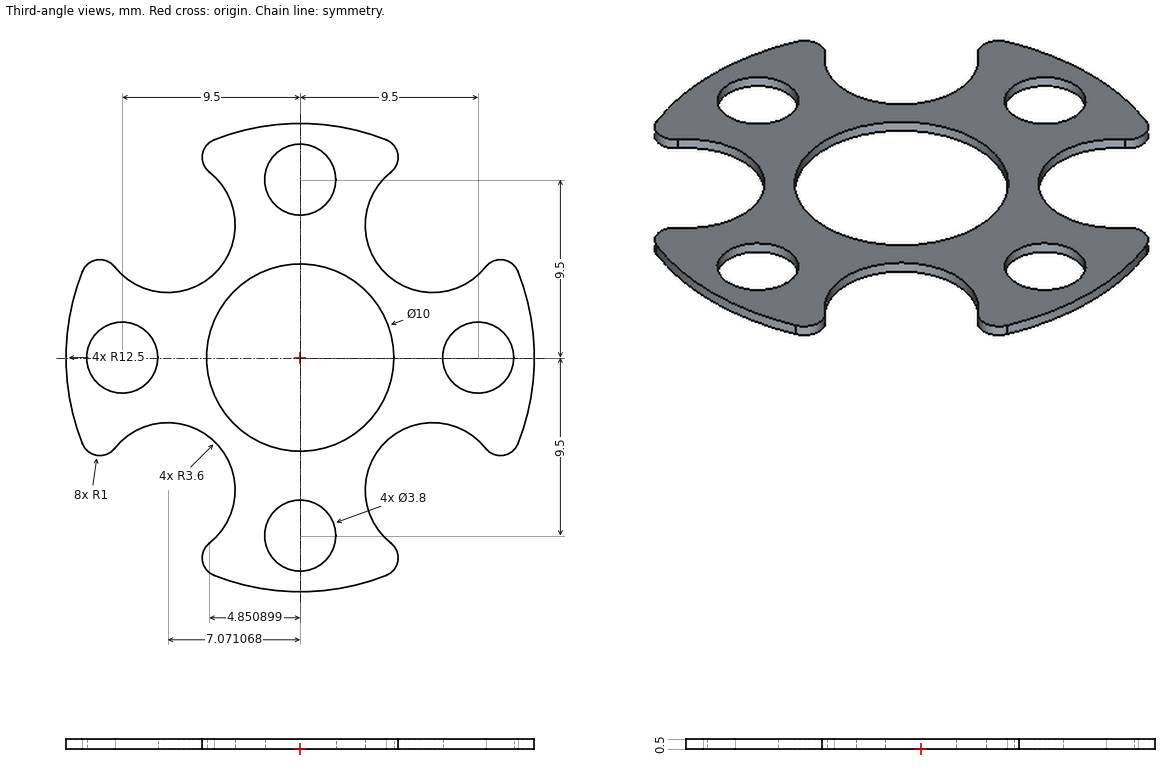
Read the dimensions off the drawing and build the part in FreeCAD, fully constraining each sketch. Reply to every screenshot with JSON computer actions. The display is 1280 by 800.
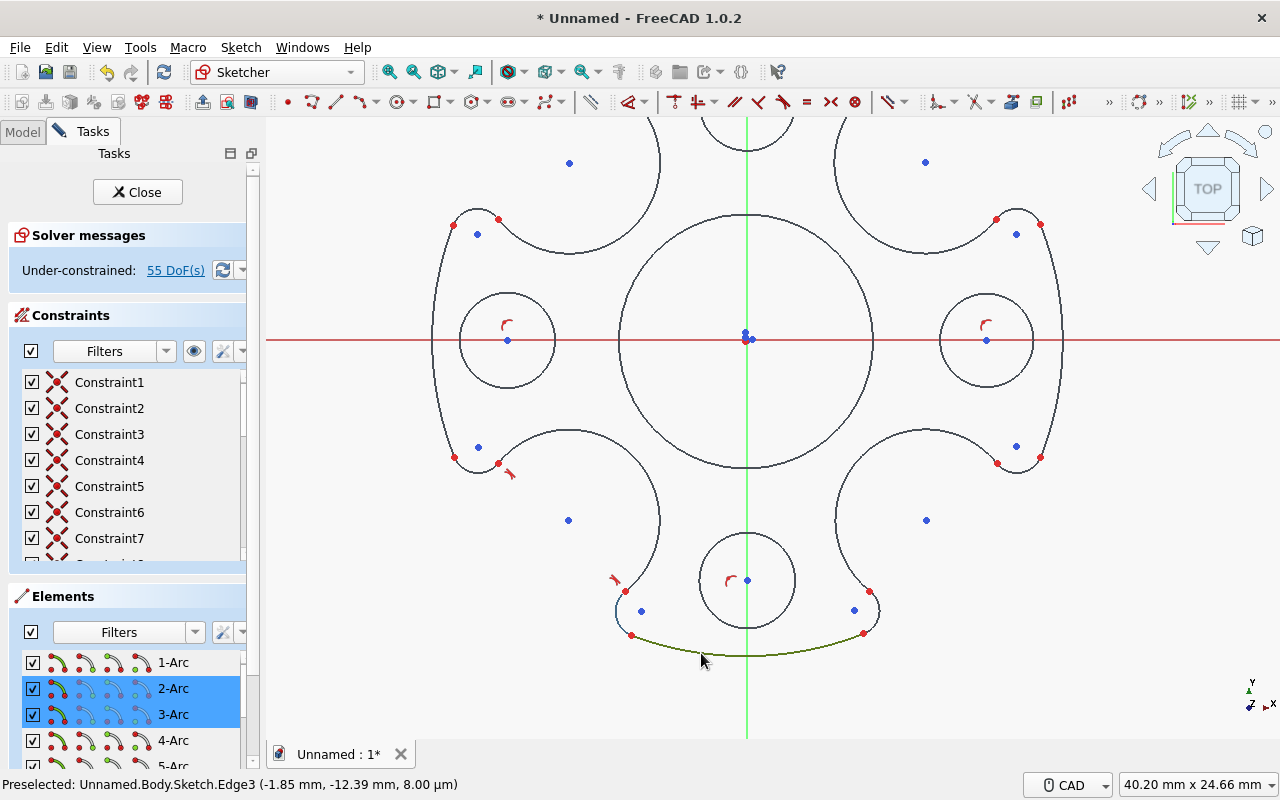
{"action": "left_click", "coordinate": [784, 102]}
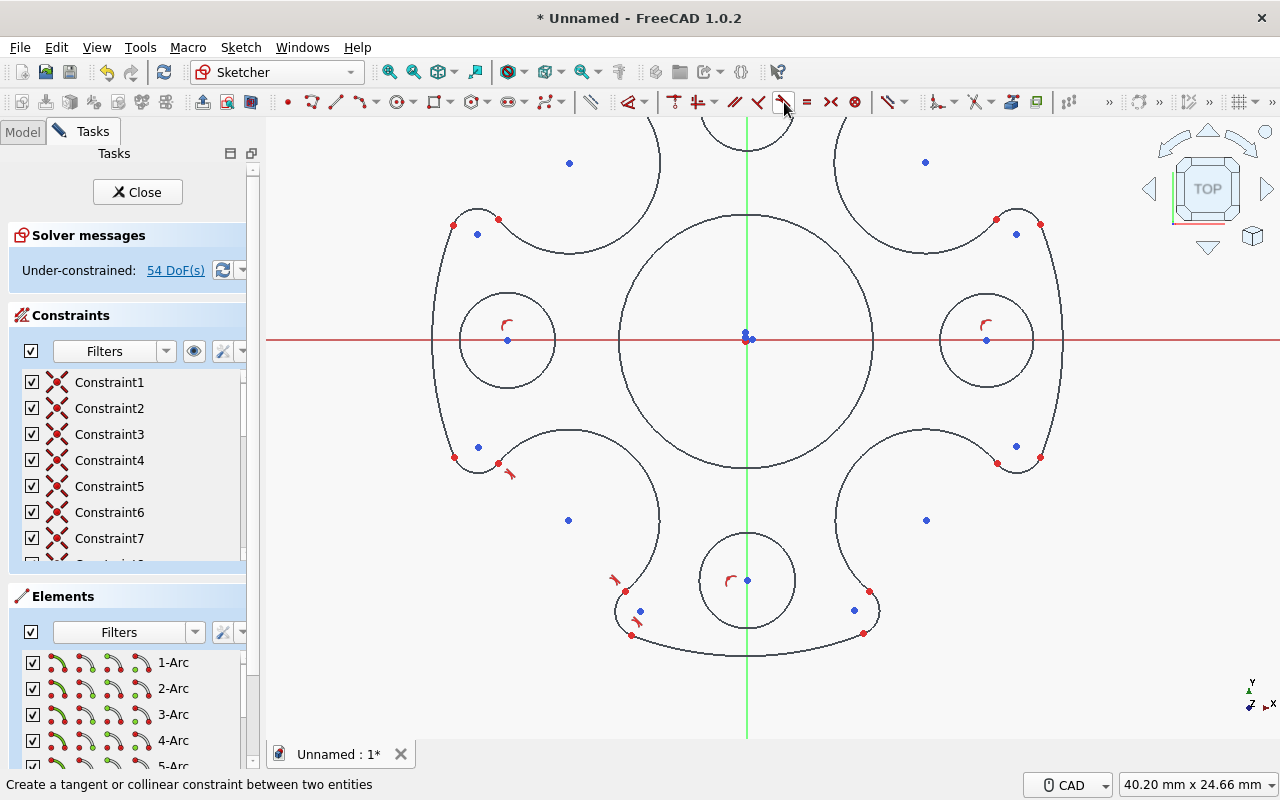
{"action": "left_click", "coordinate": [701, 653]}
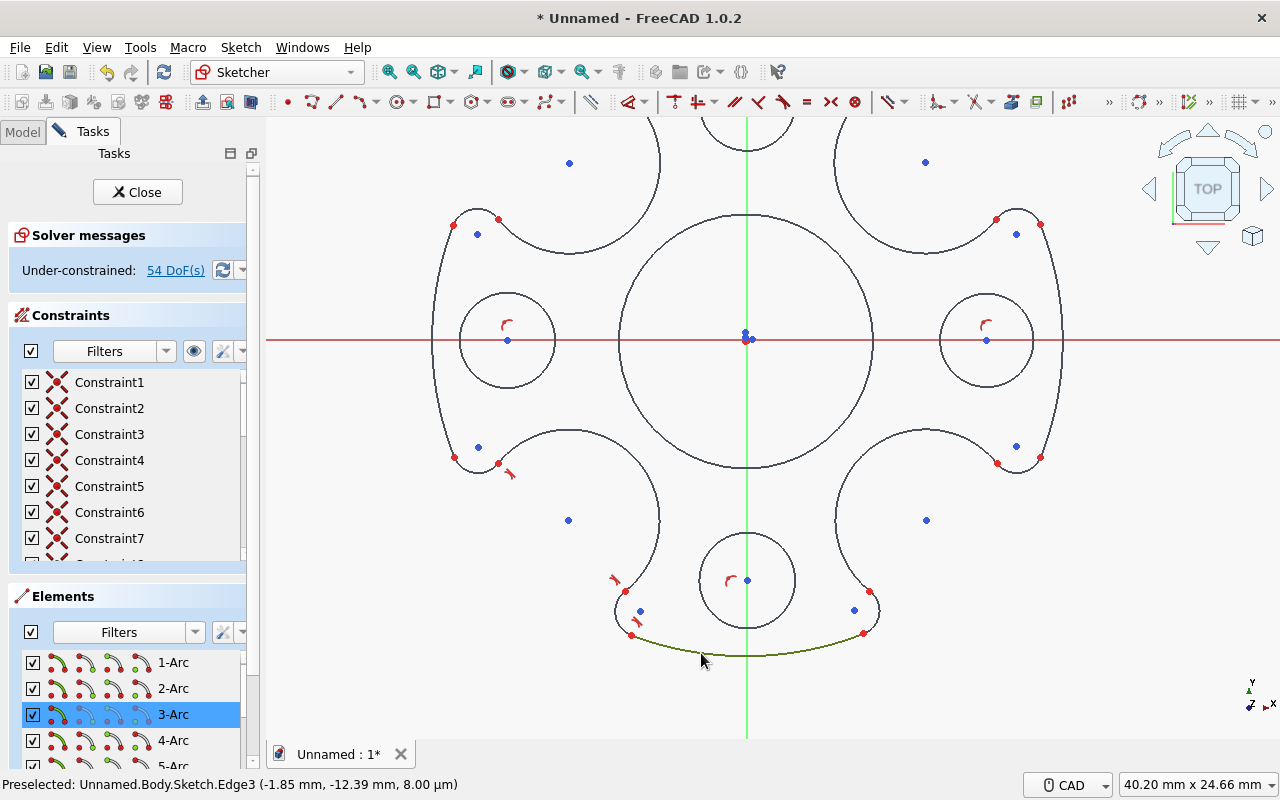
{"action": "left_click", "coordinate": [875, 624]}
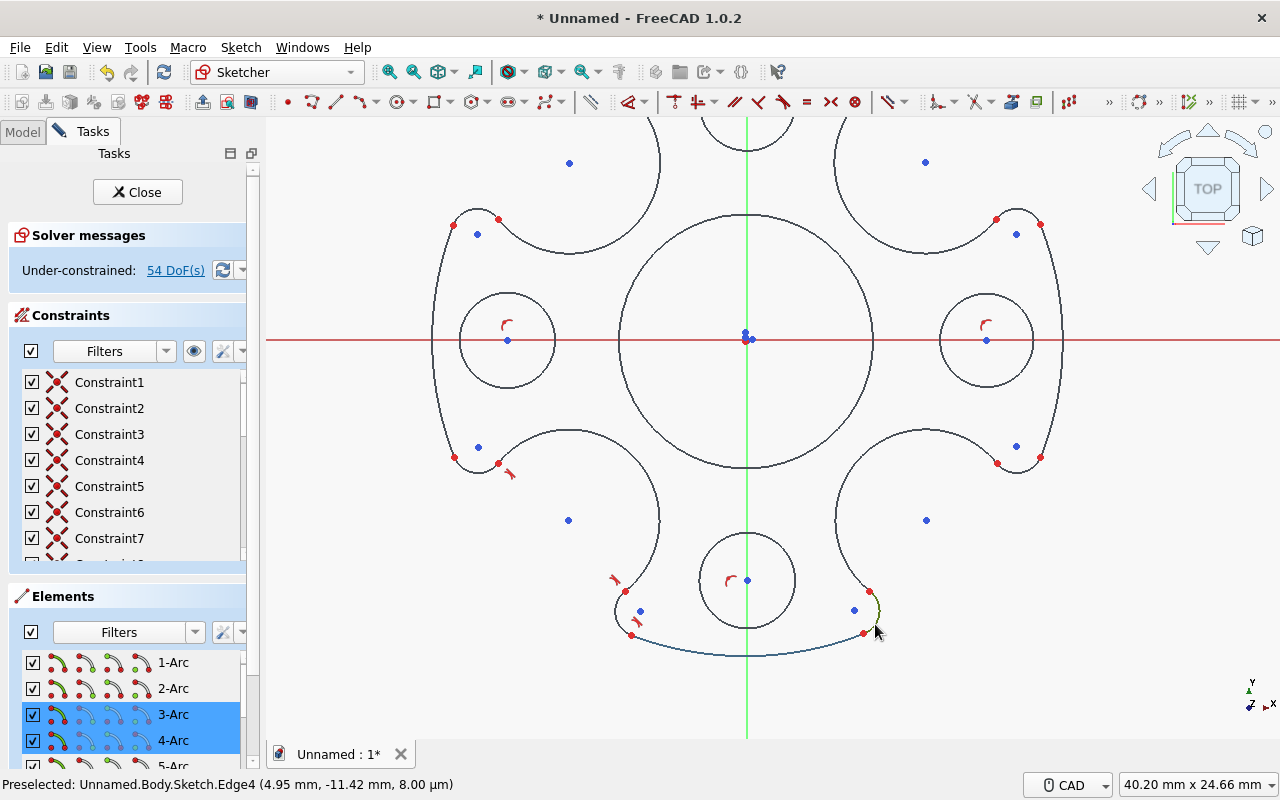
{"action": "key", "text": "t"}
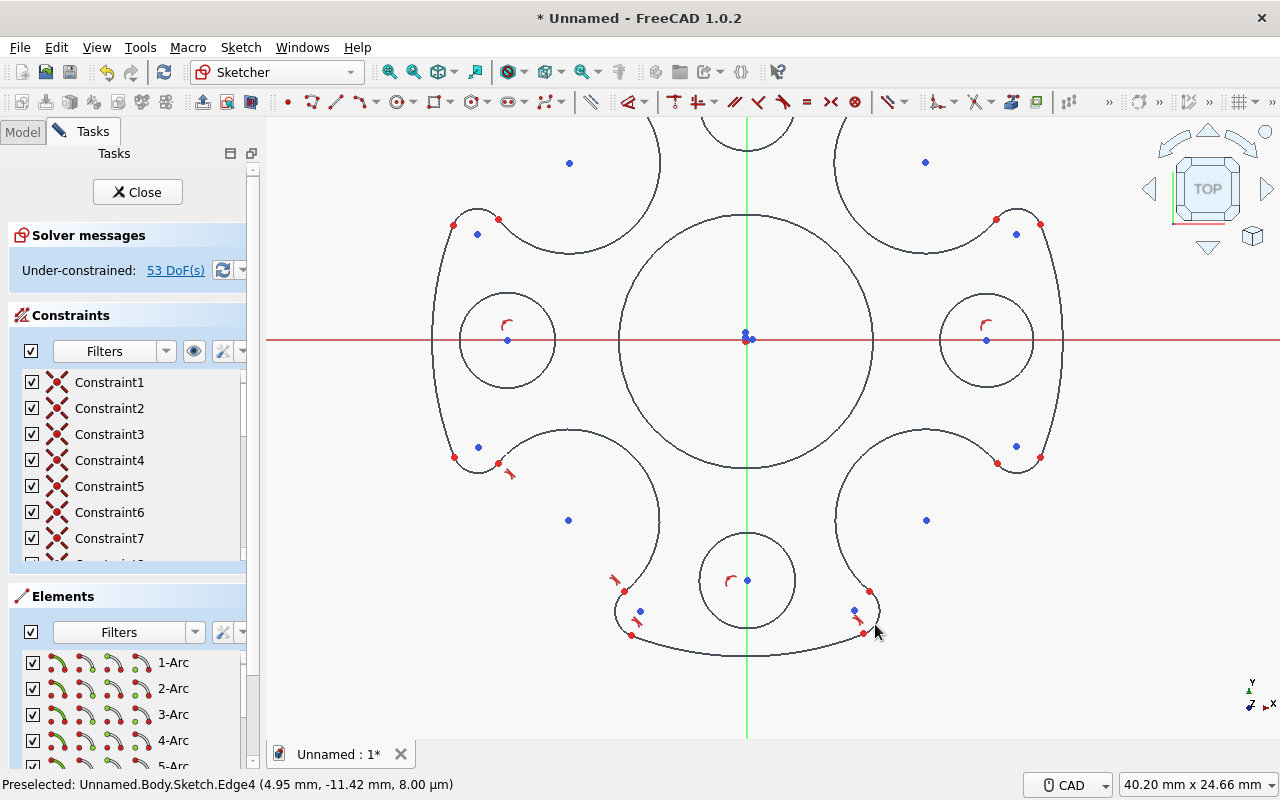
{"action": "left_click", "coordinate": [876, 624]}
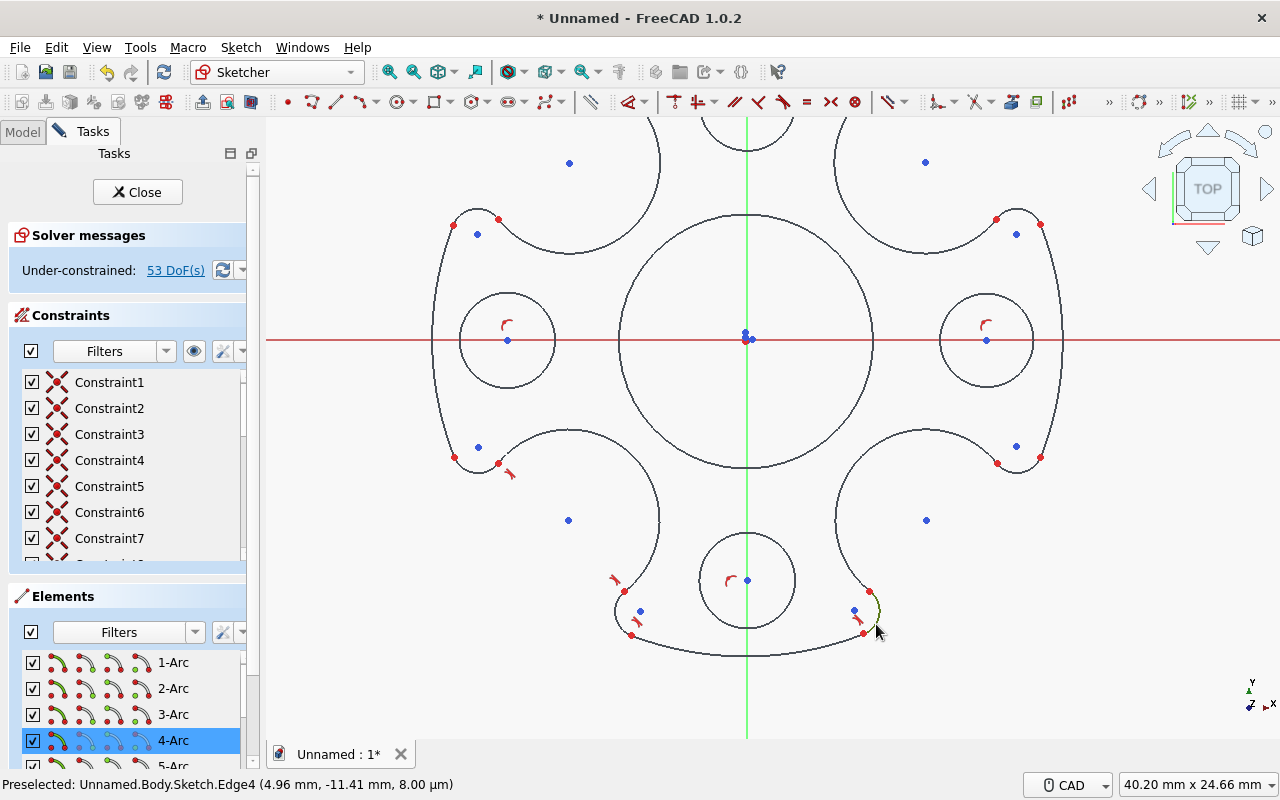
{"action": "left_click", "coordinate": [916, 430]}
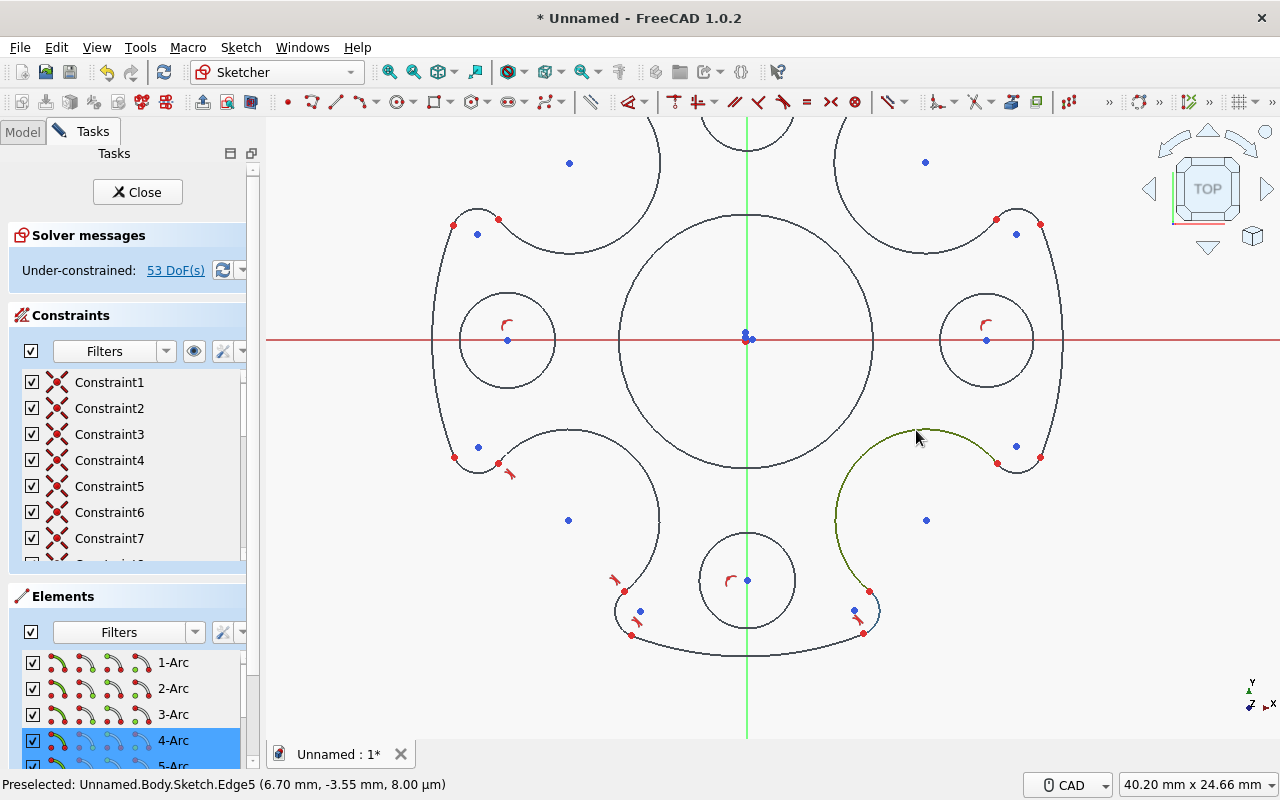
{"action": "key", "text": "t"}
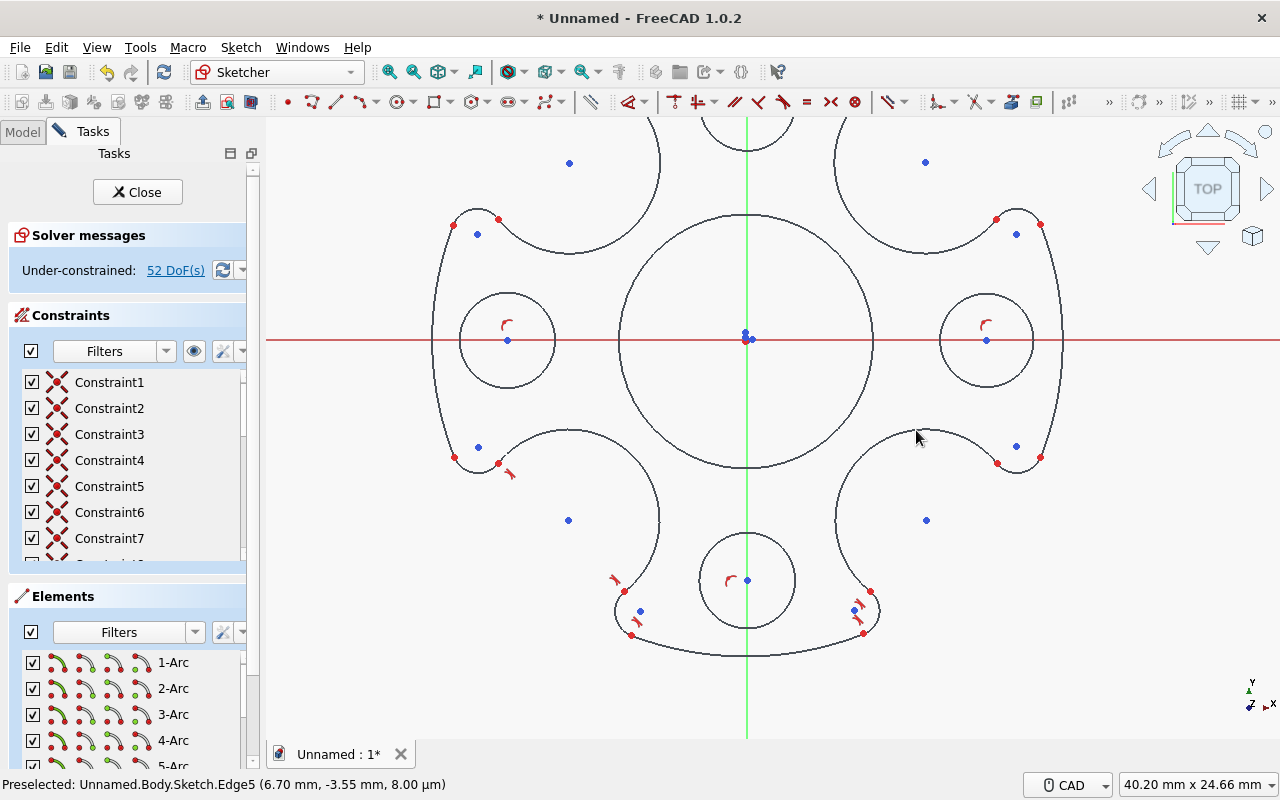
{"action": "left_click", "coordinate": [916, 430]}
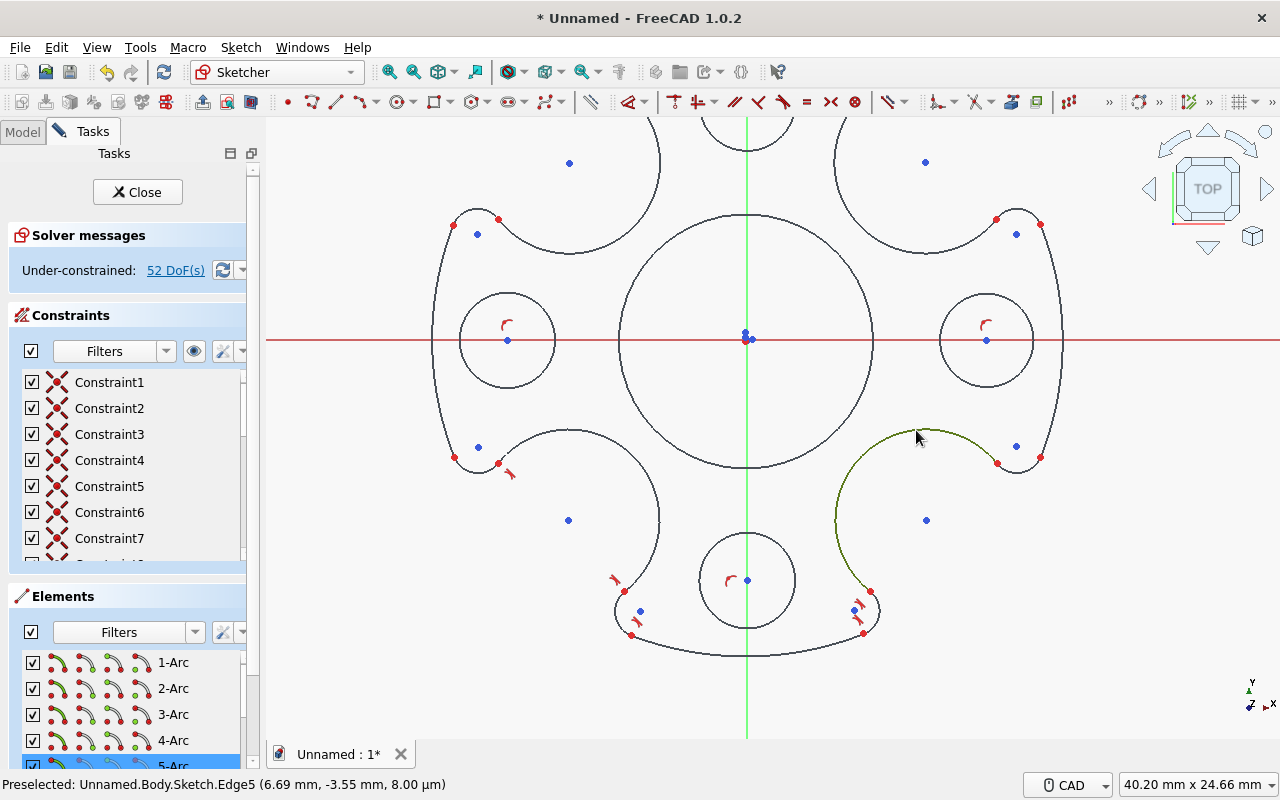
{"action": "left_click", "coordinate": [1010, 472]}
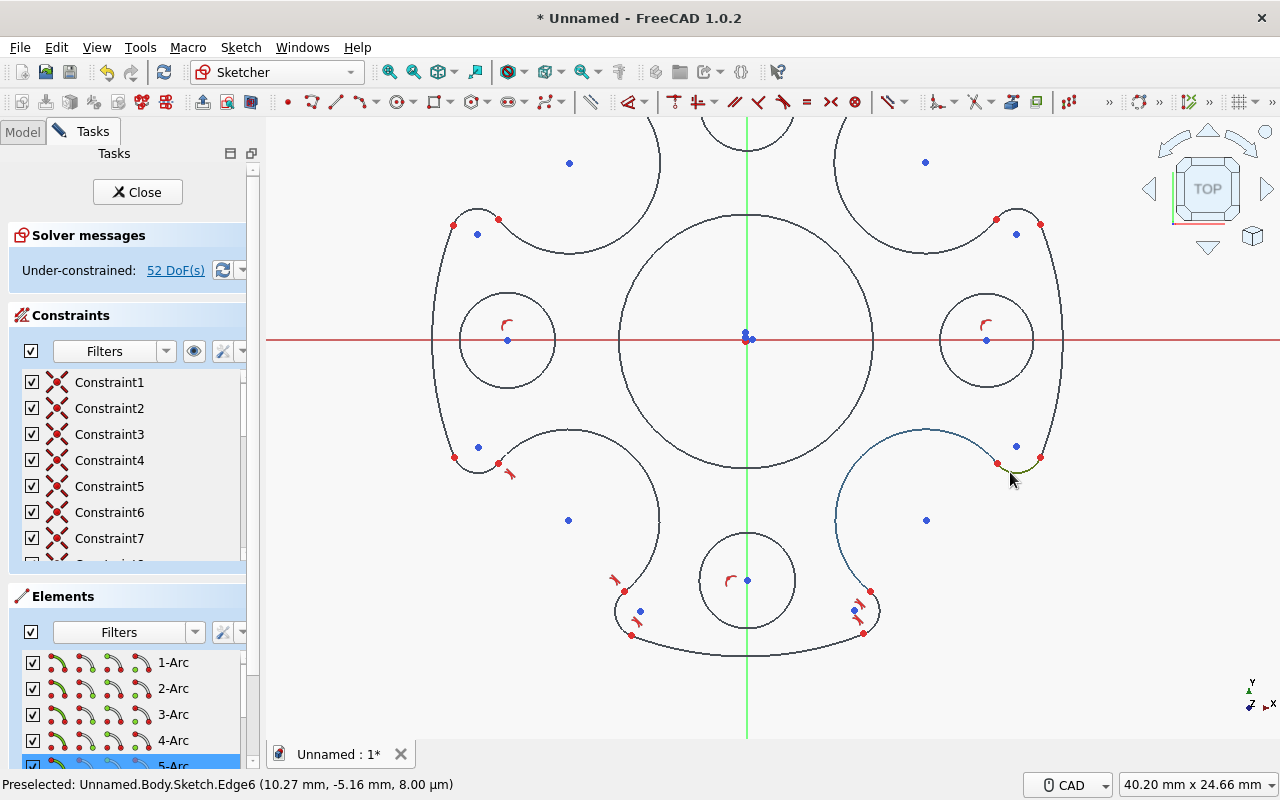
{"action": "key", "text": "t"}